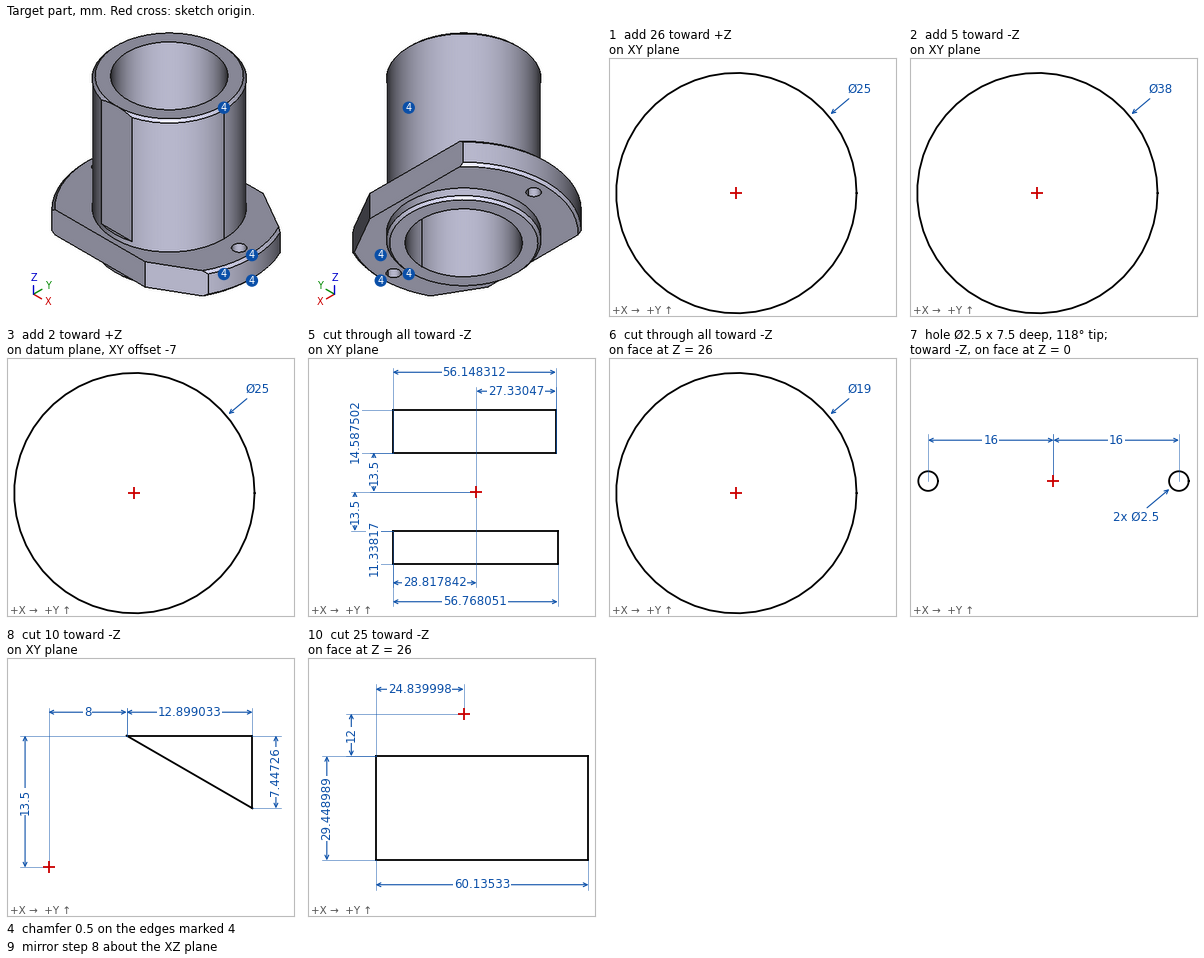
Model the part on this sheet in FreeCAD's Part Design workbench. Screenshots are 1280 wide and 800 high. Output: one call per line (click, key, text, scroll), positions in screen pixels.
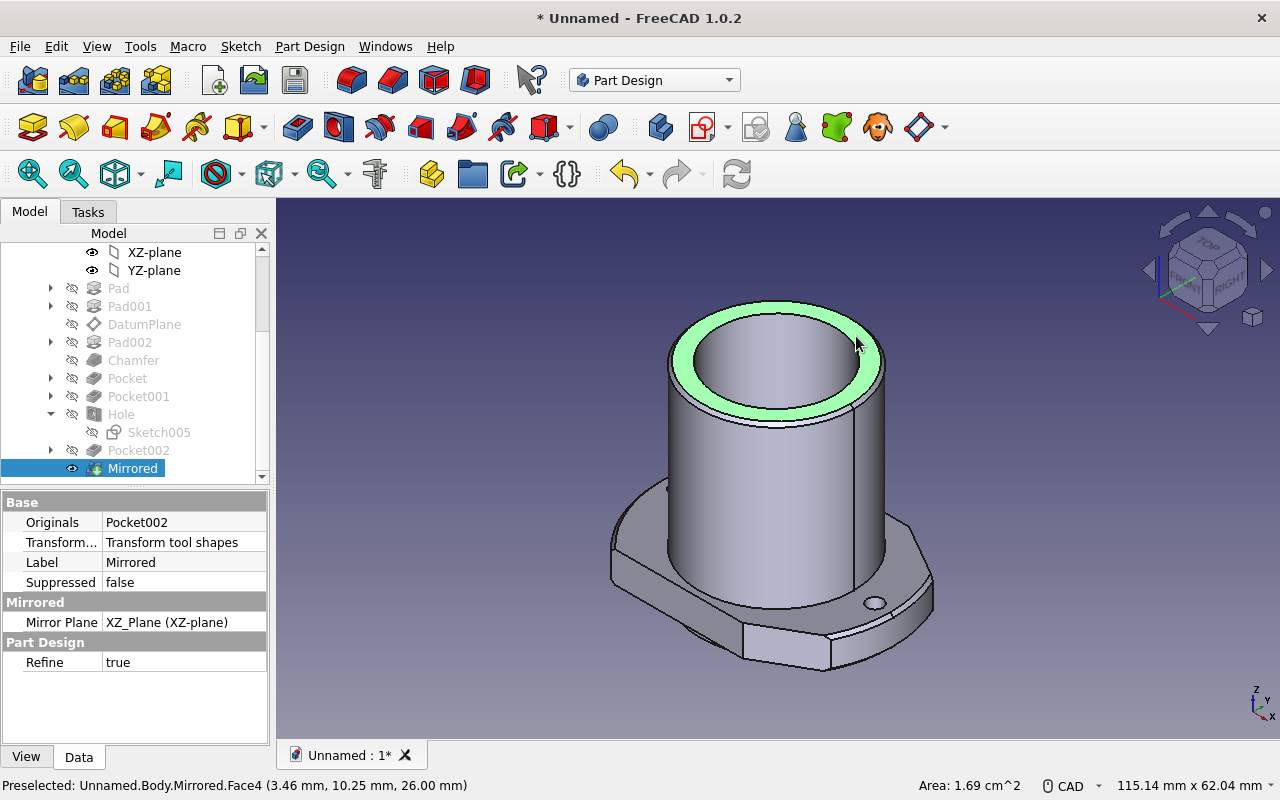
click(702, 128)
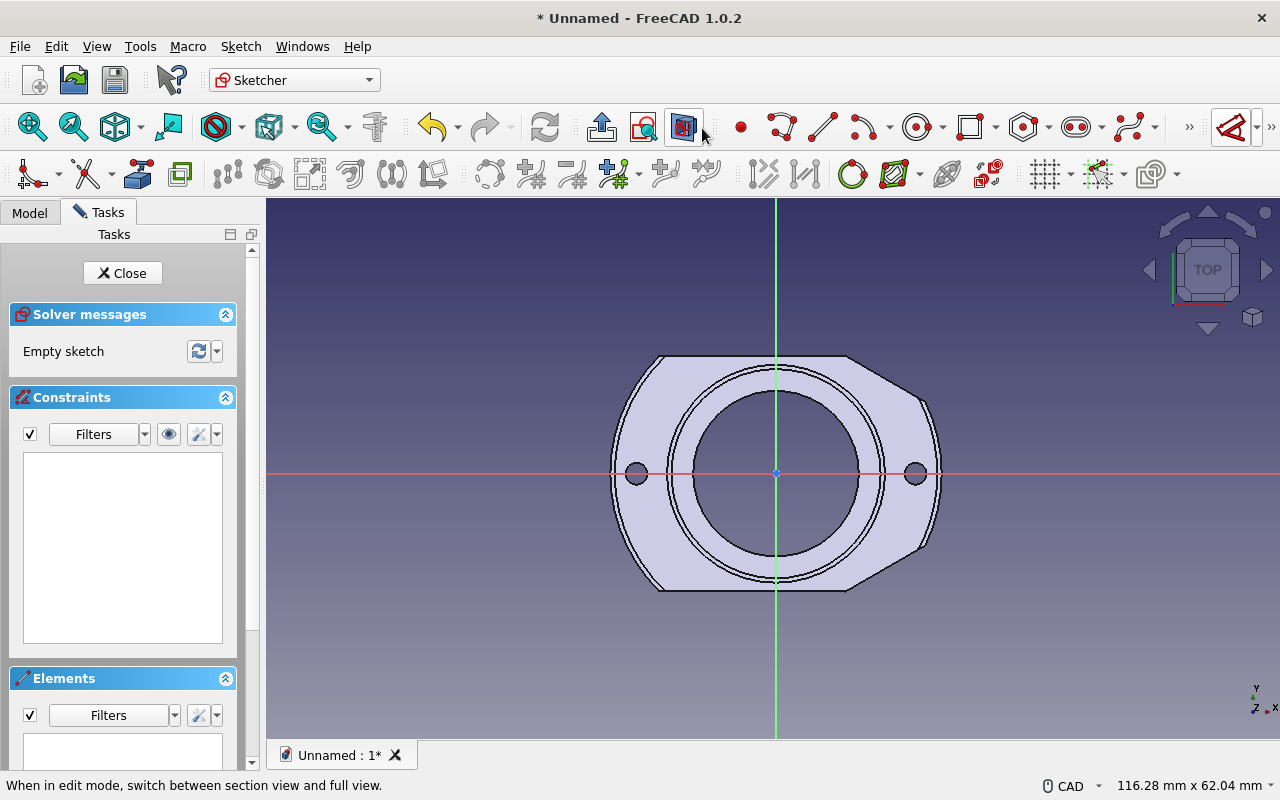
scroll(466, 226, down, 2)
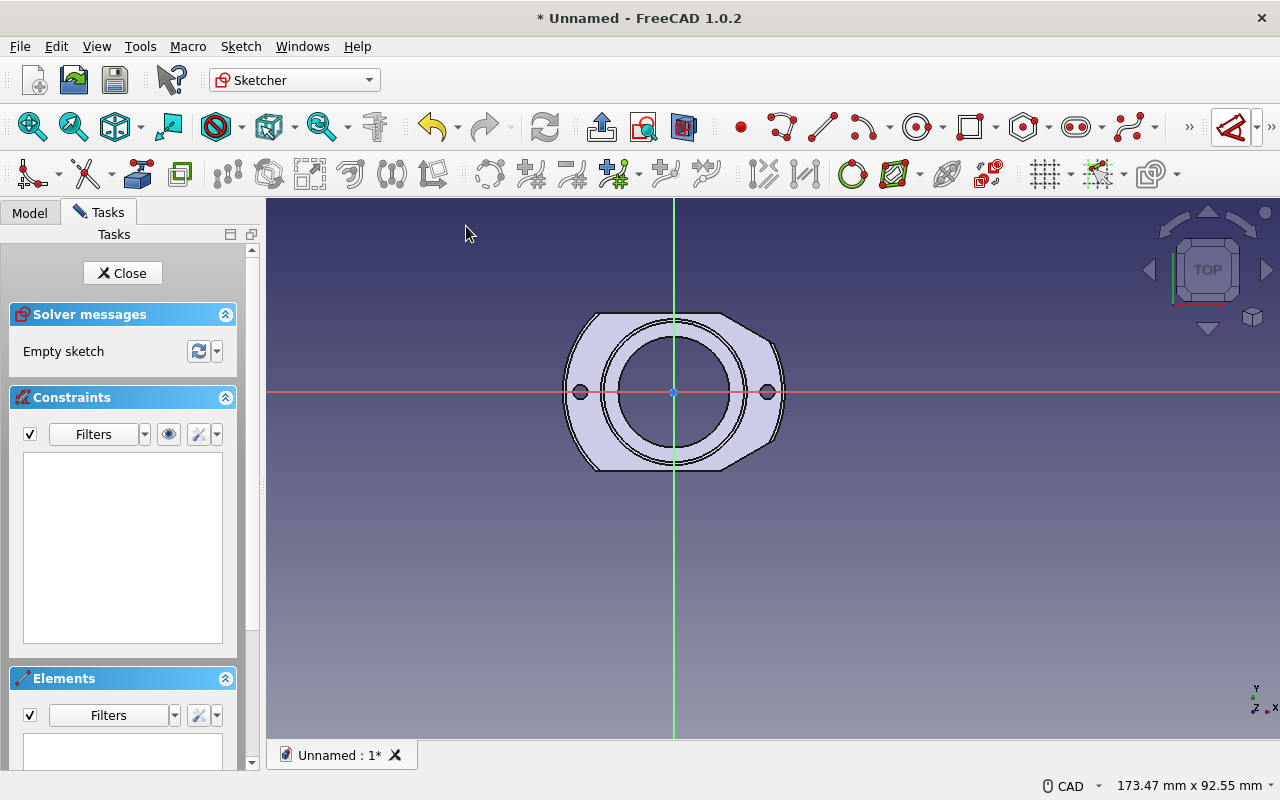
scroll(704, 604, up, 2)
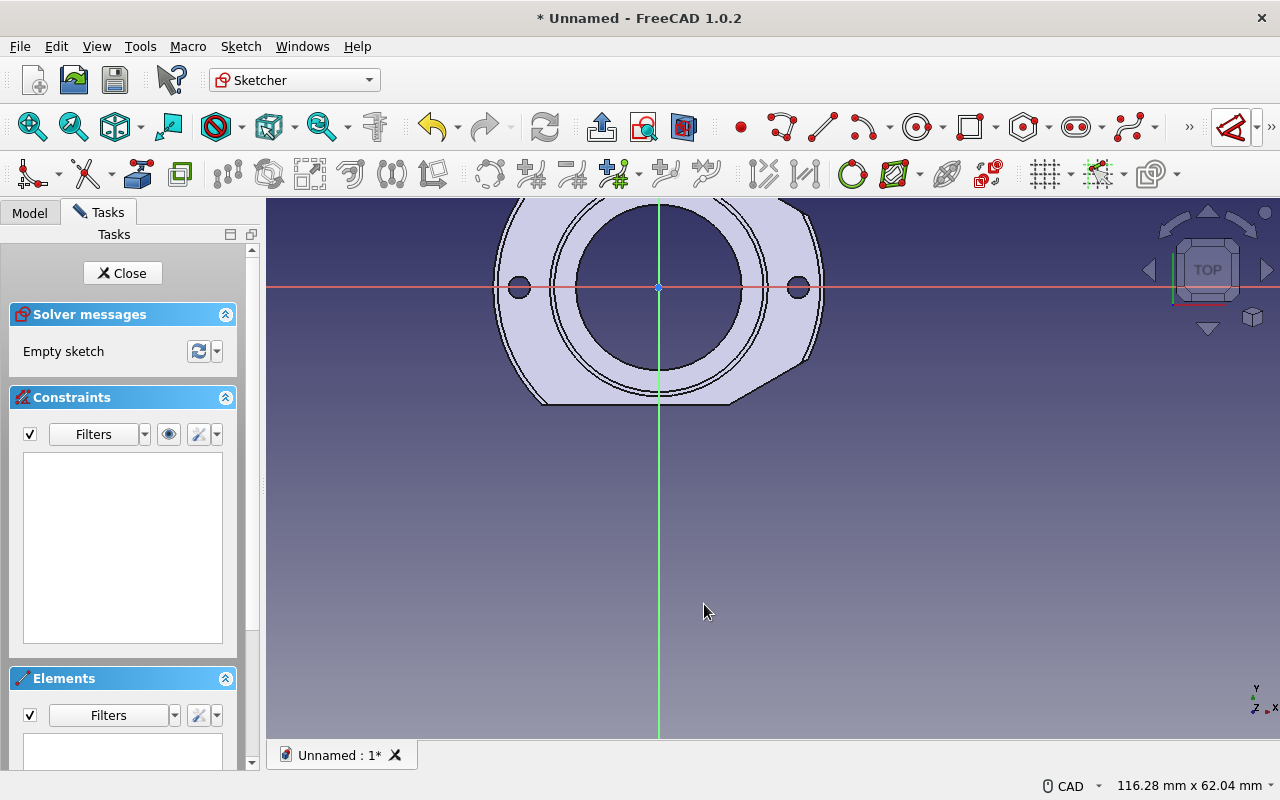
click(970, 128)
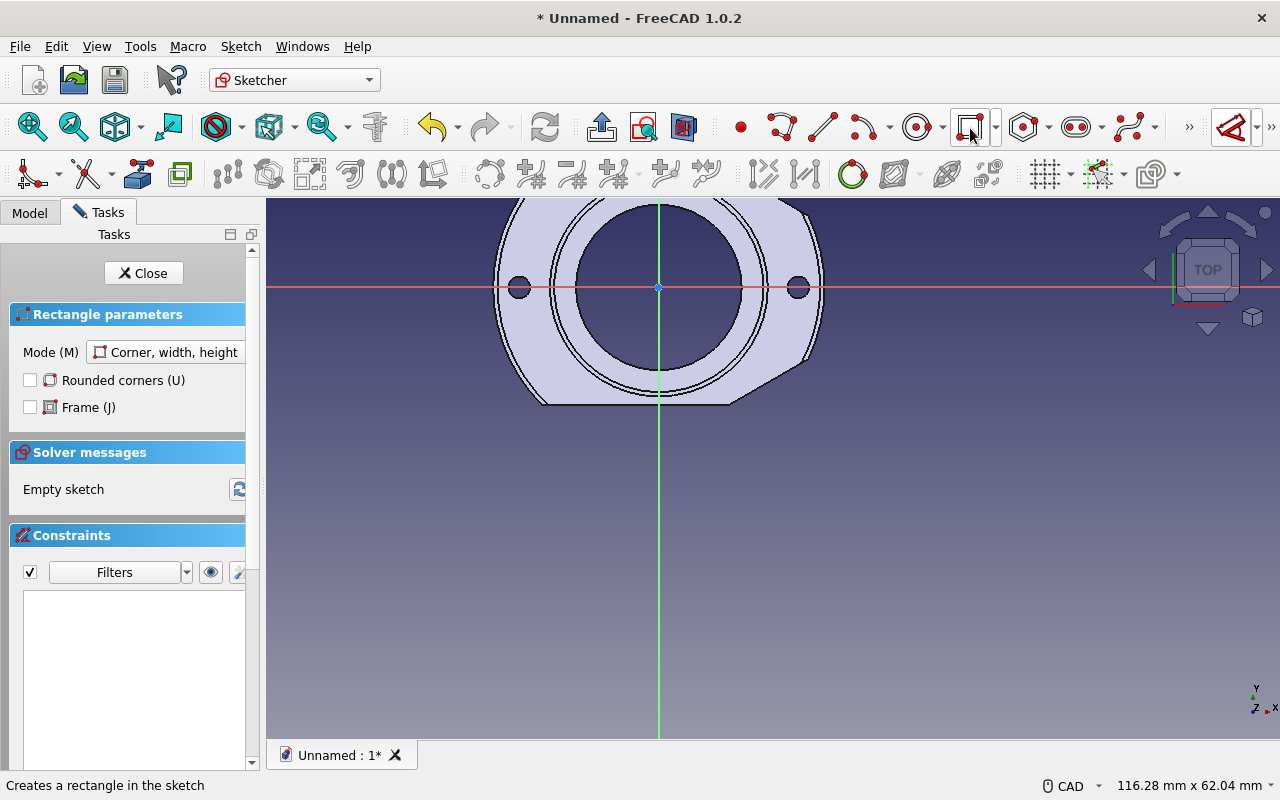
click(442, 392)
click(967, 649)
key(Escape)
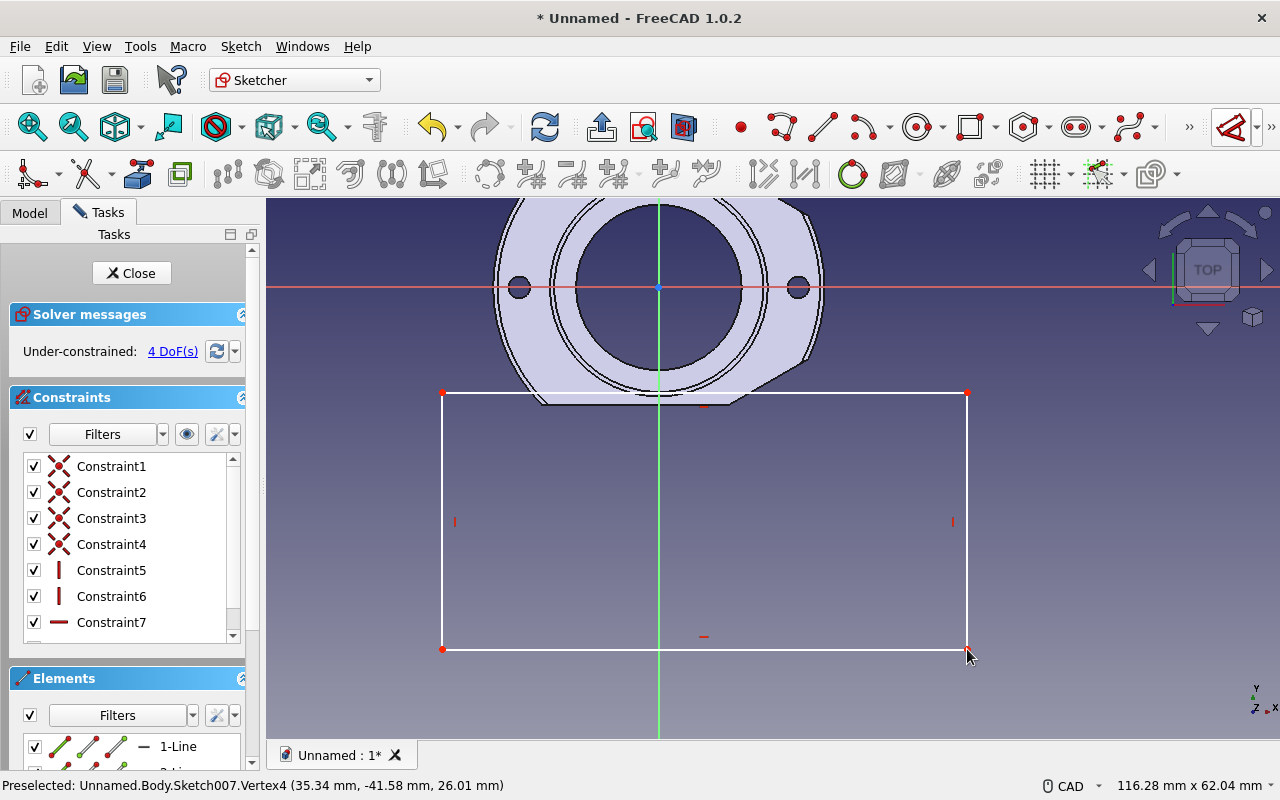
click(442, 393)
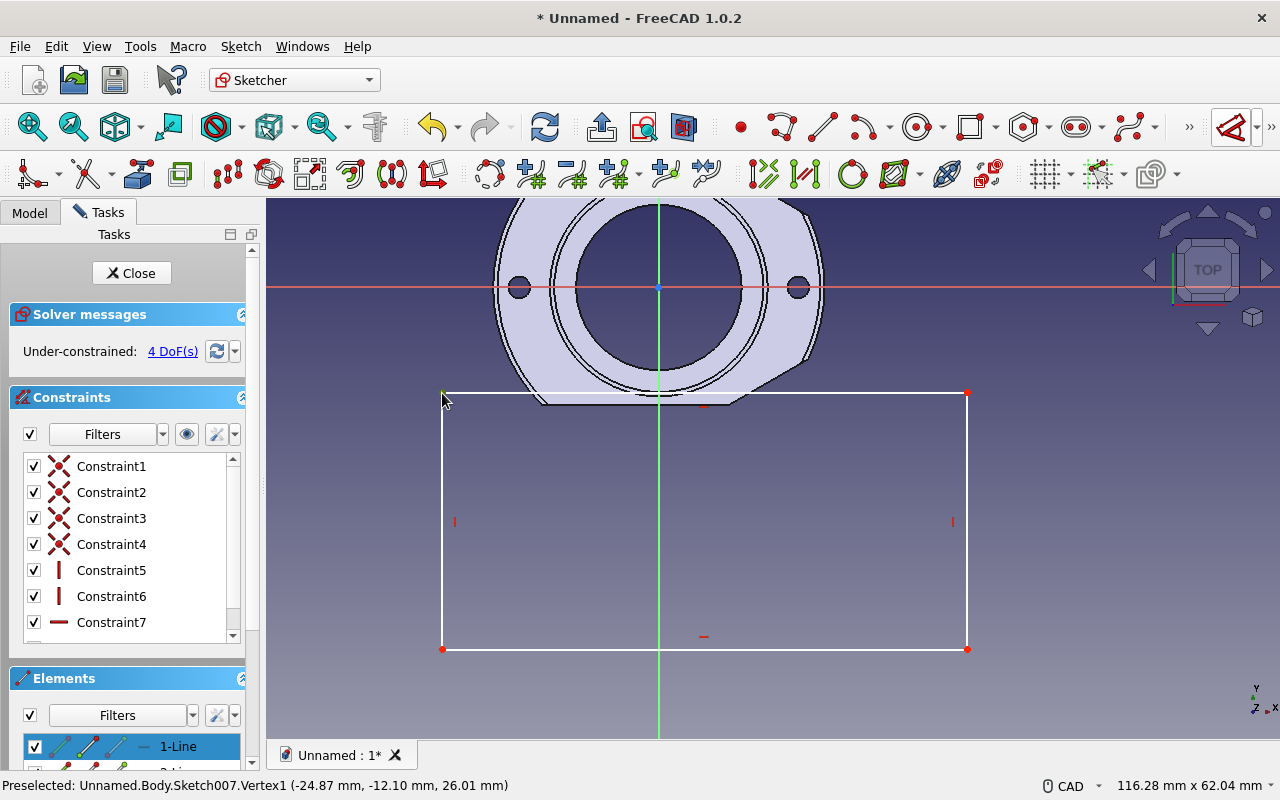
key(i)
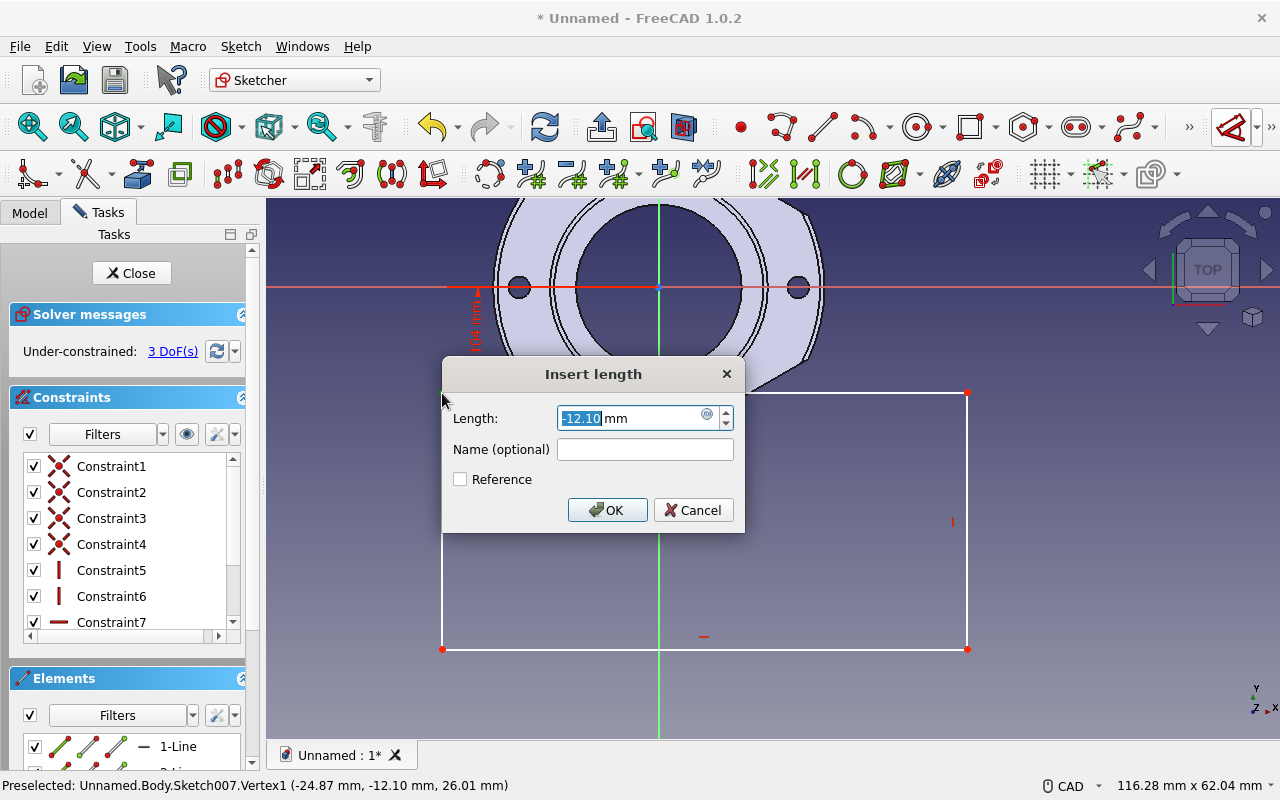
text(-12)
key(Return)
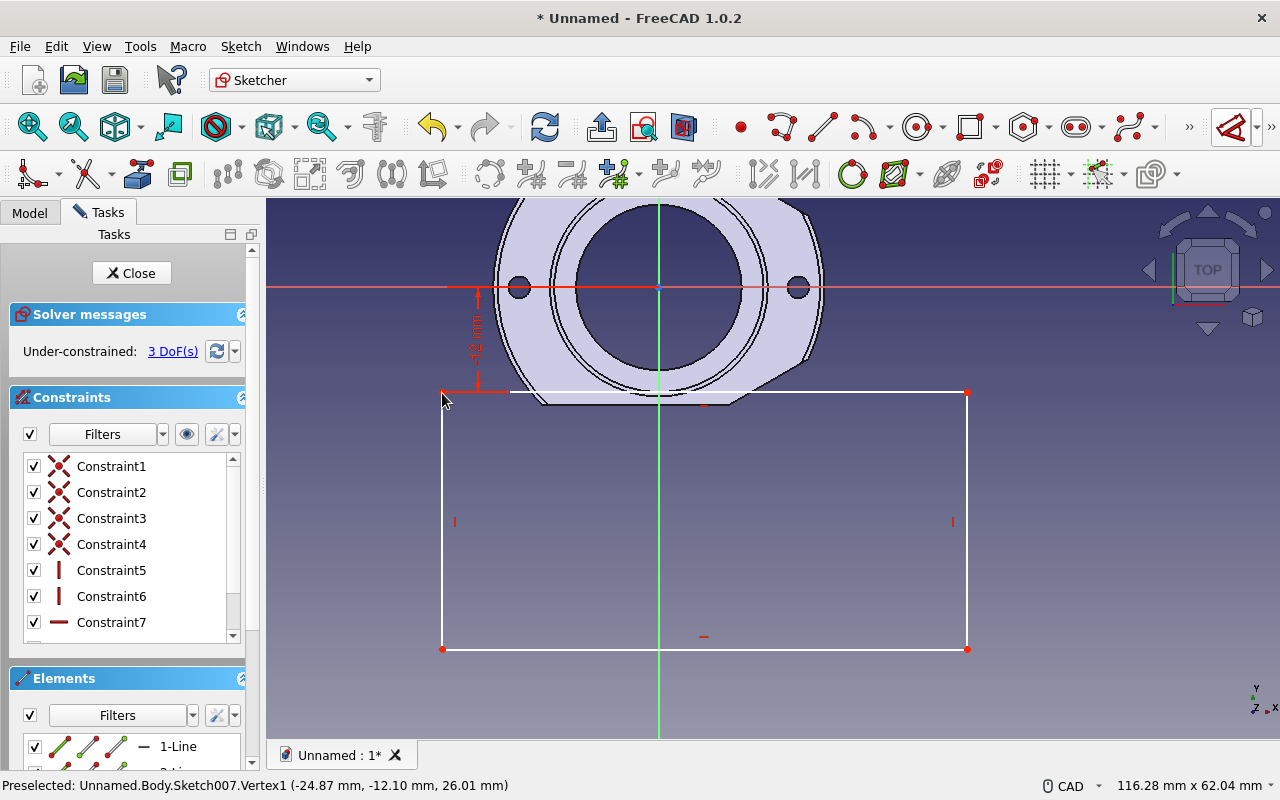
click(600, 650)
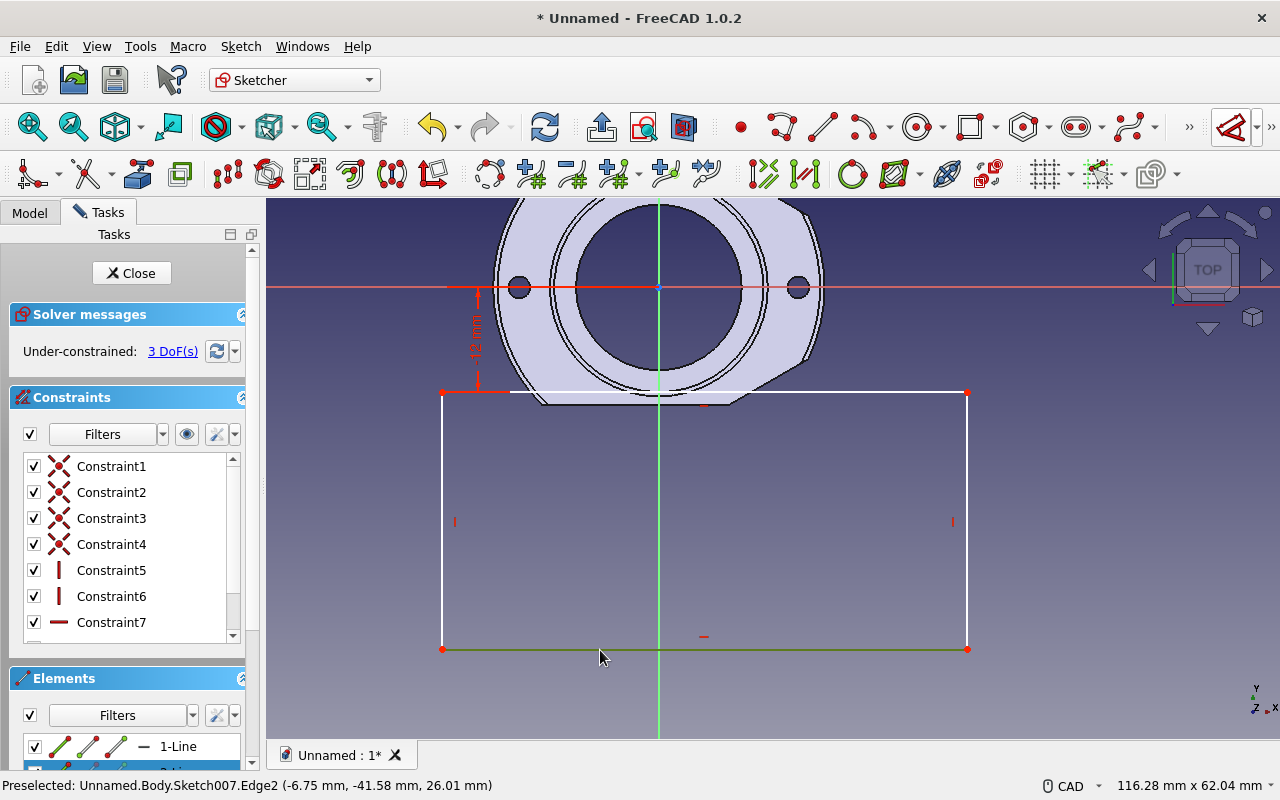
click(1256, 128)